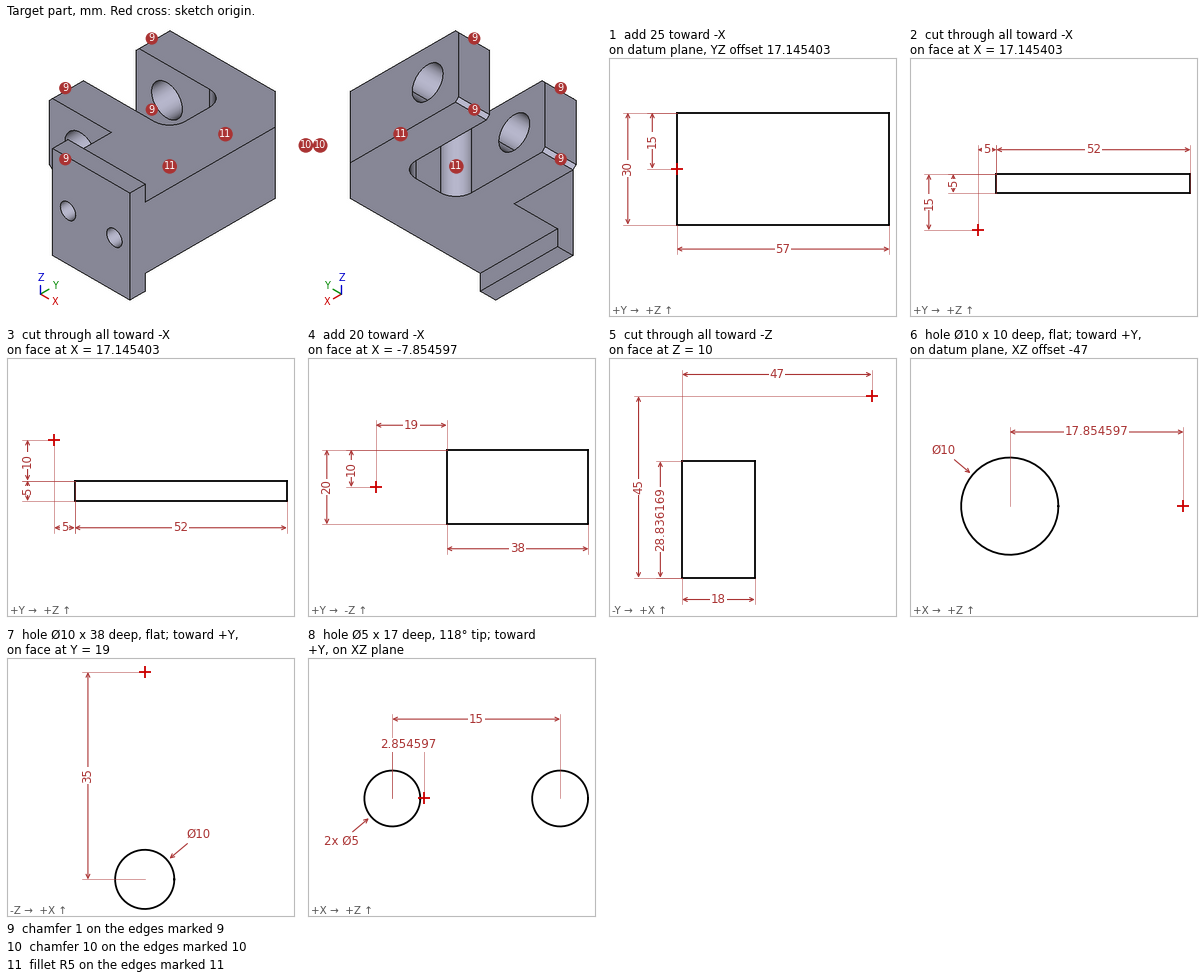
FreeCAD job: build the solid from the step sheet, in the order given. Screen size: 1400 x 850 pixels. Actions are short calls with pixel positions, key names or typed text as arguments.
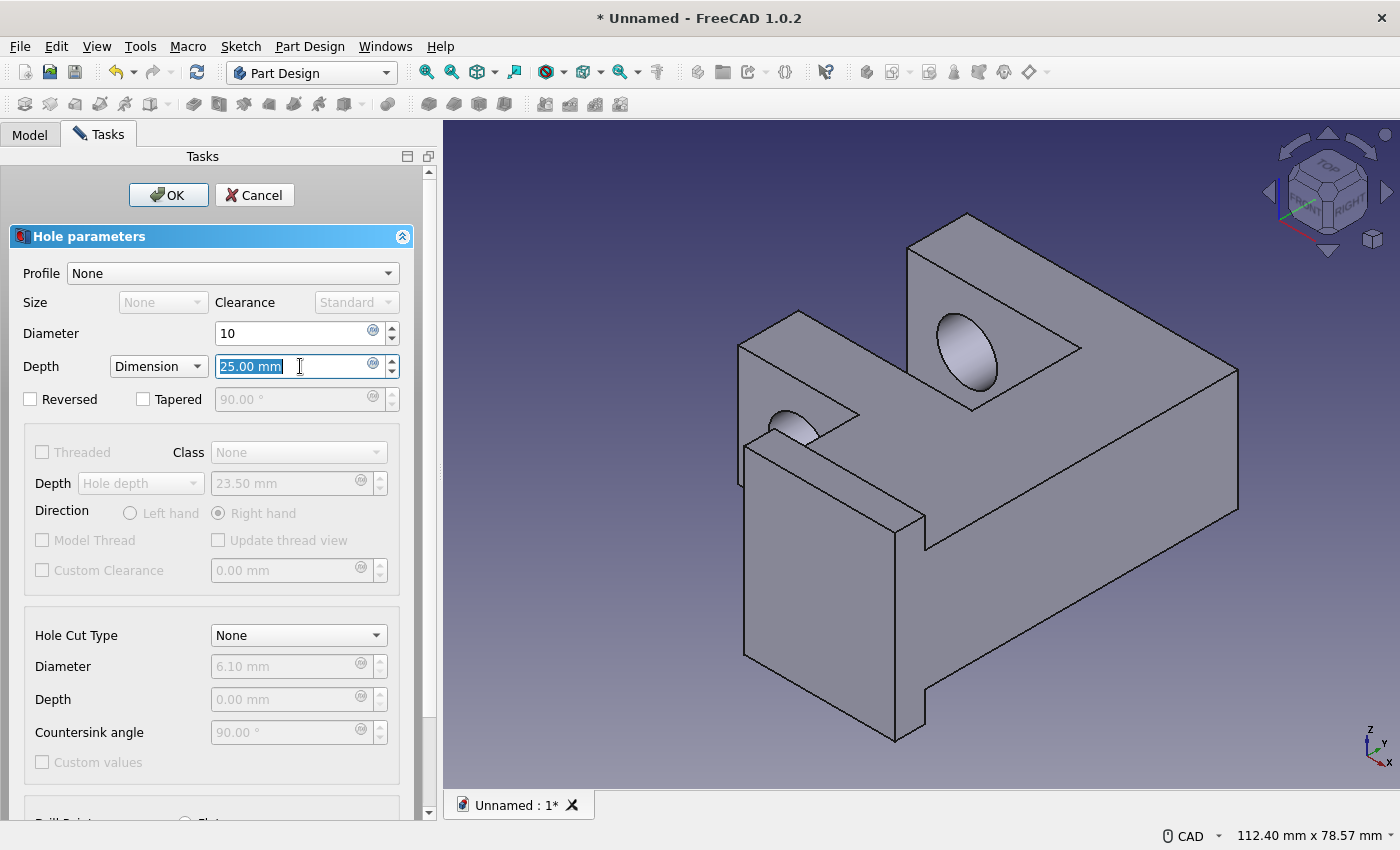
text(38)
key(Tab)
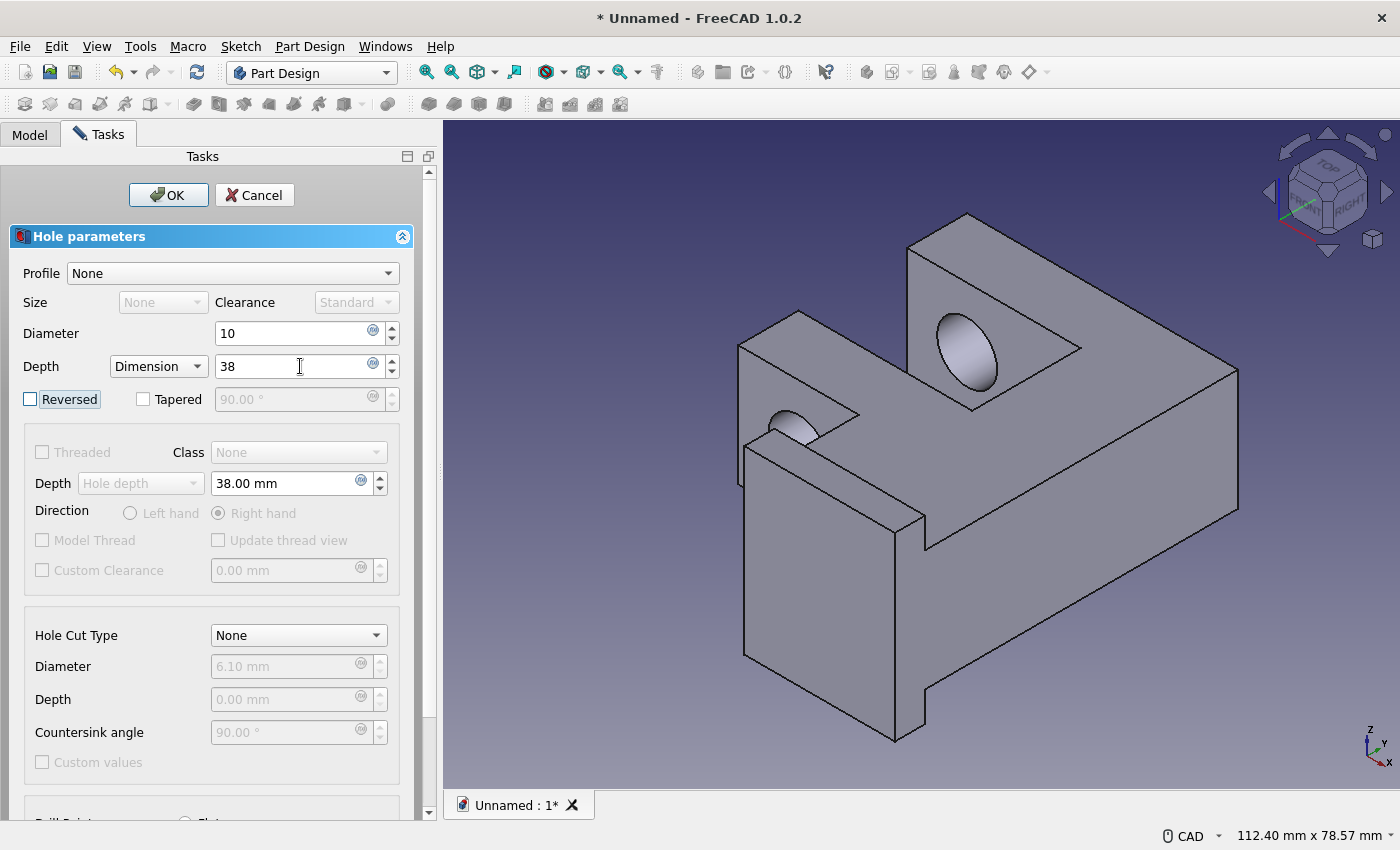
scroll(429, 493, down, 2)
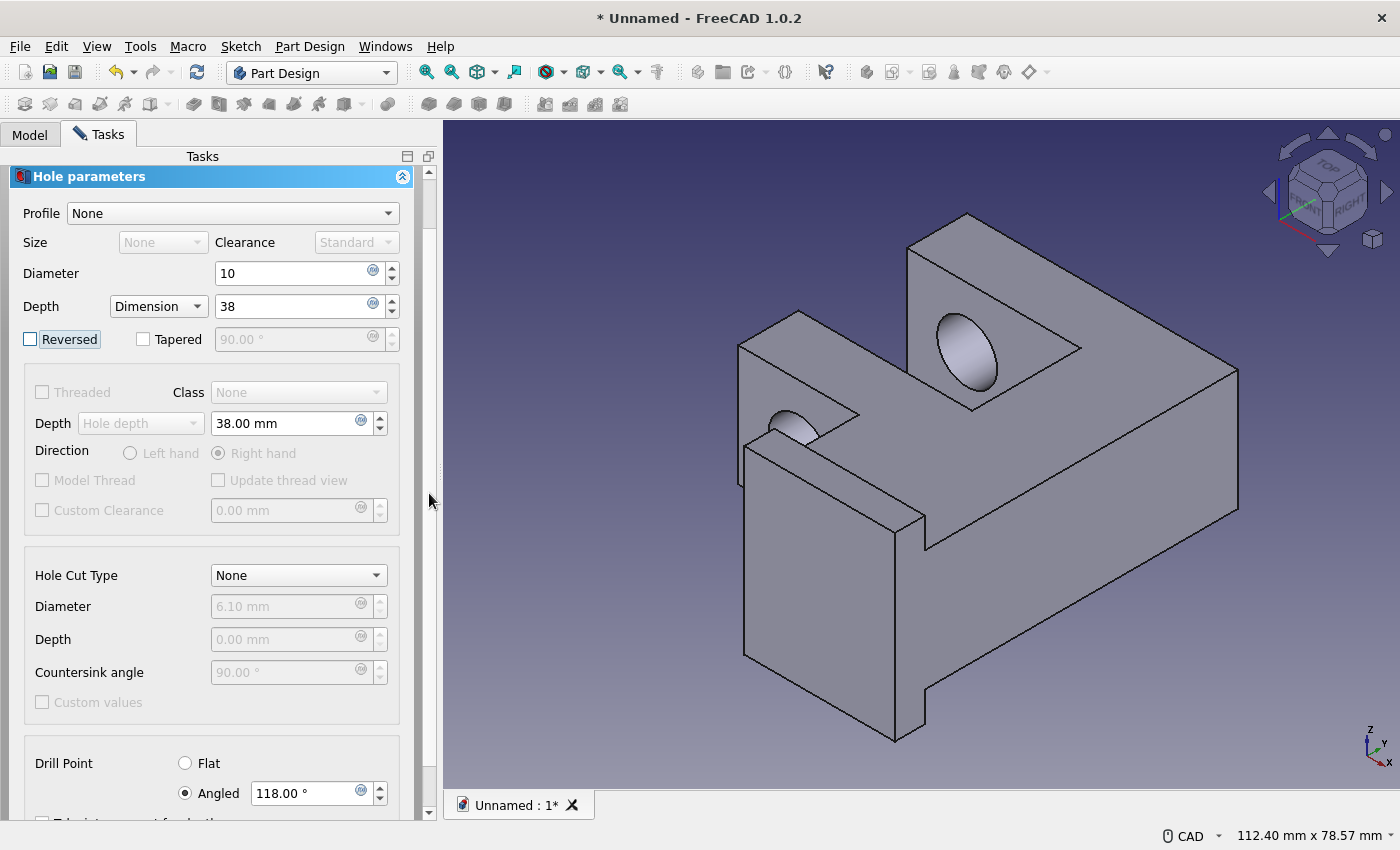
click(186, 713)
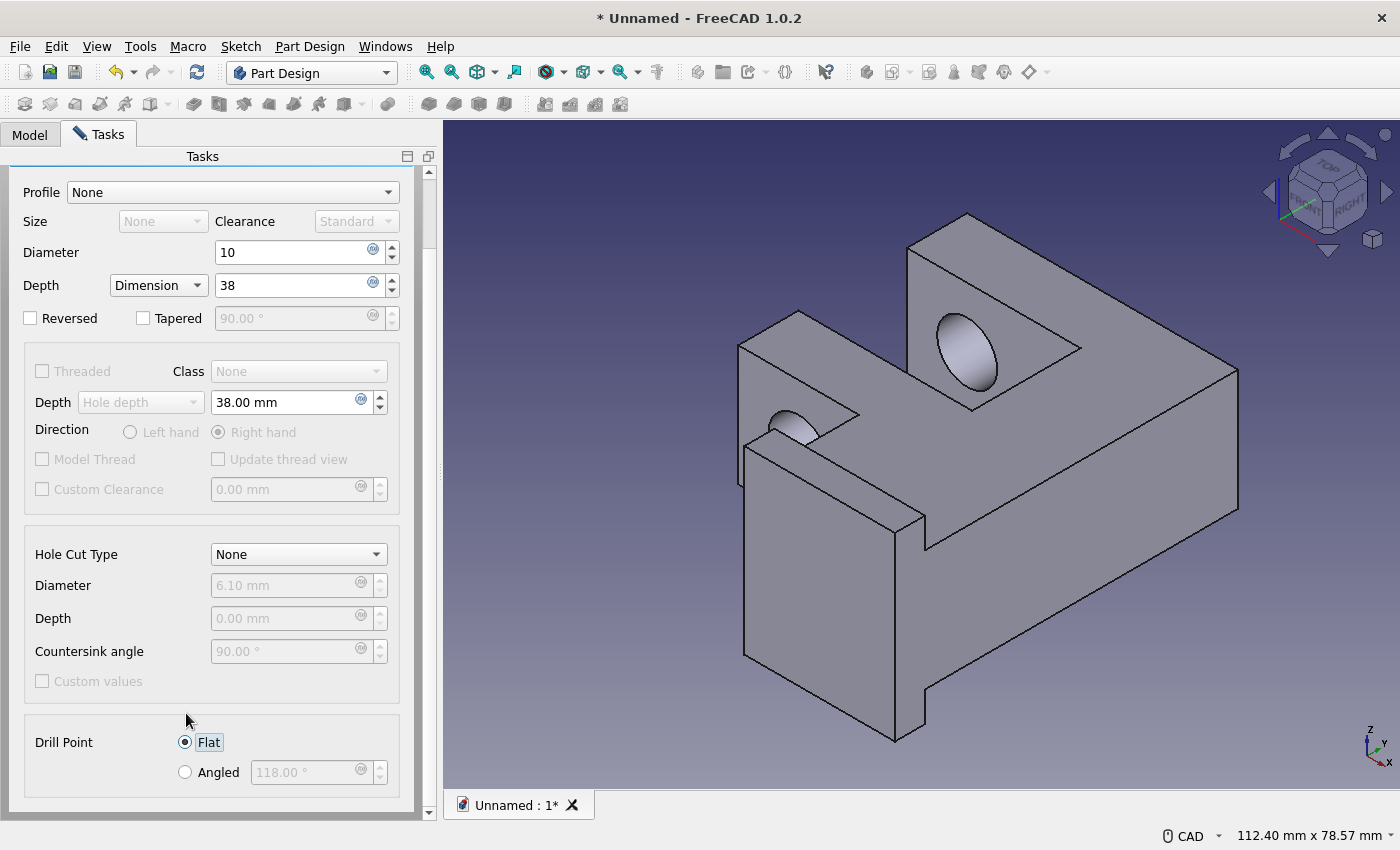
scroll(429, 493, up, 3)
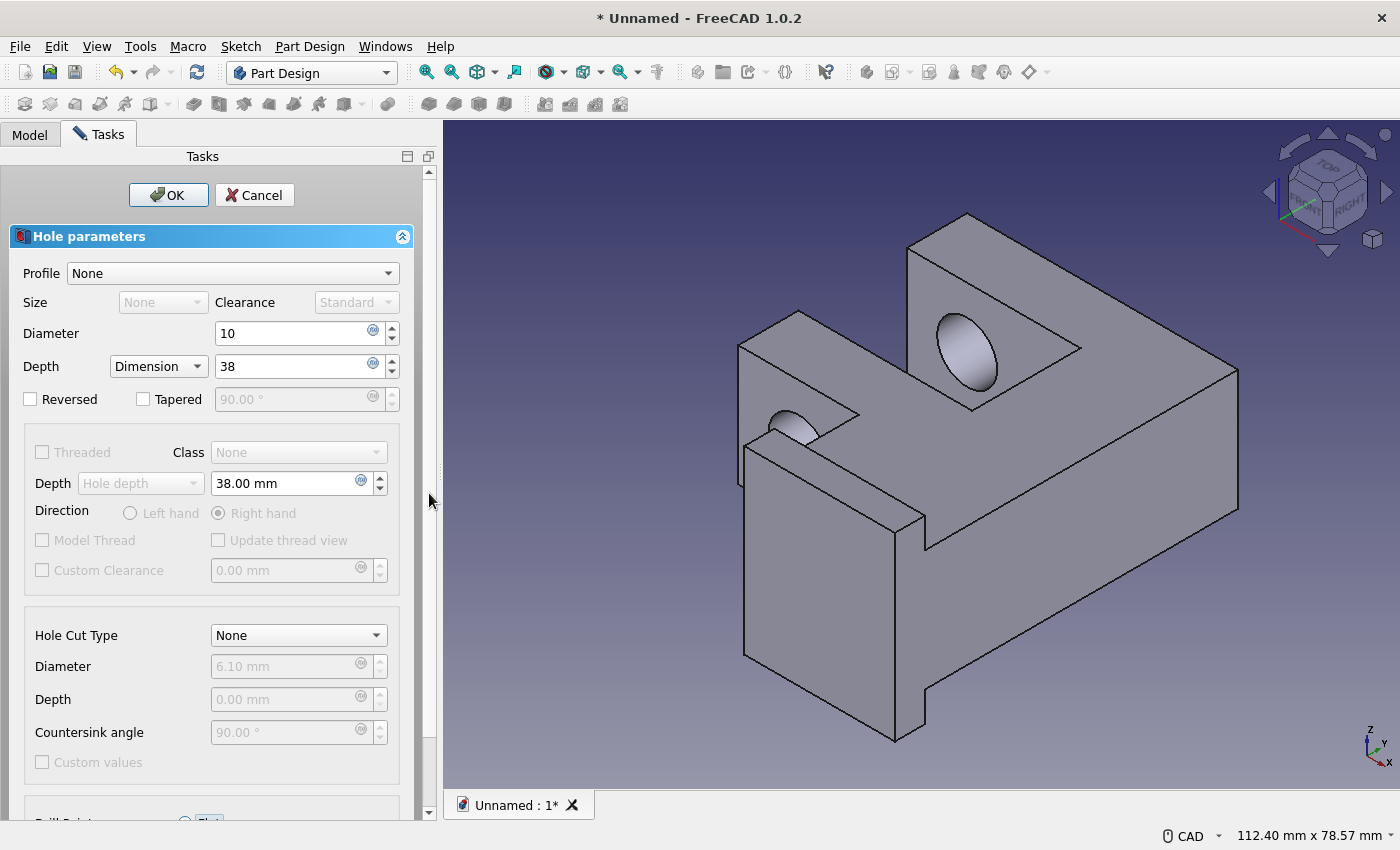
click(169, 195)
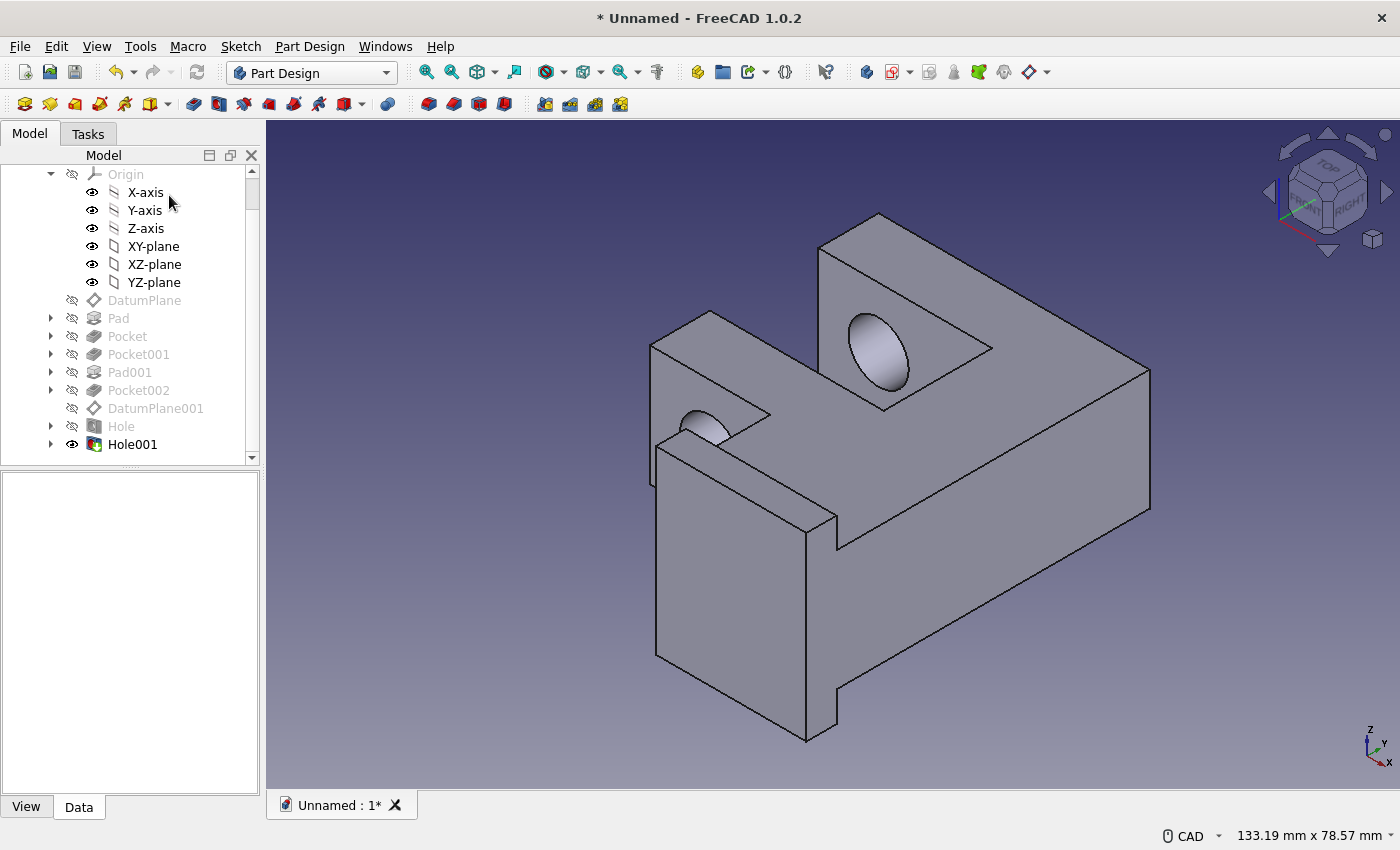
click(892, 72)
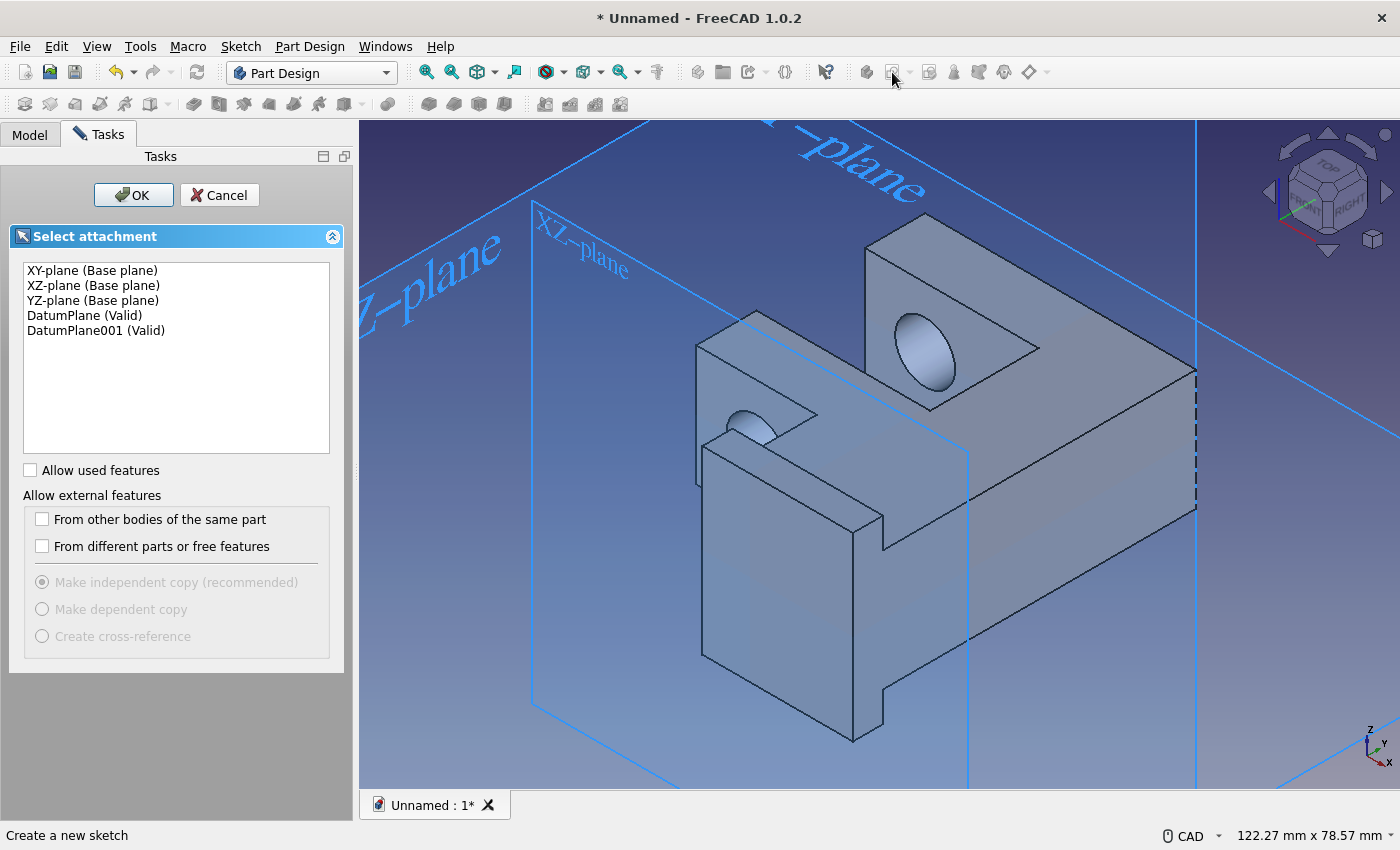
click(84, 286)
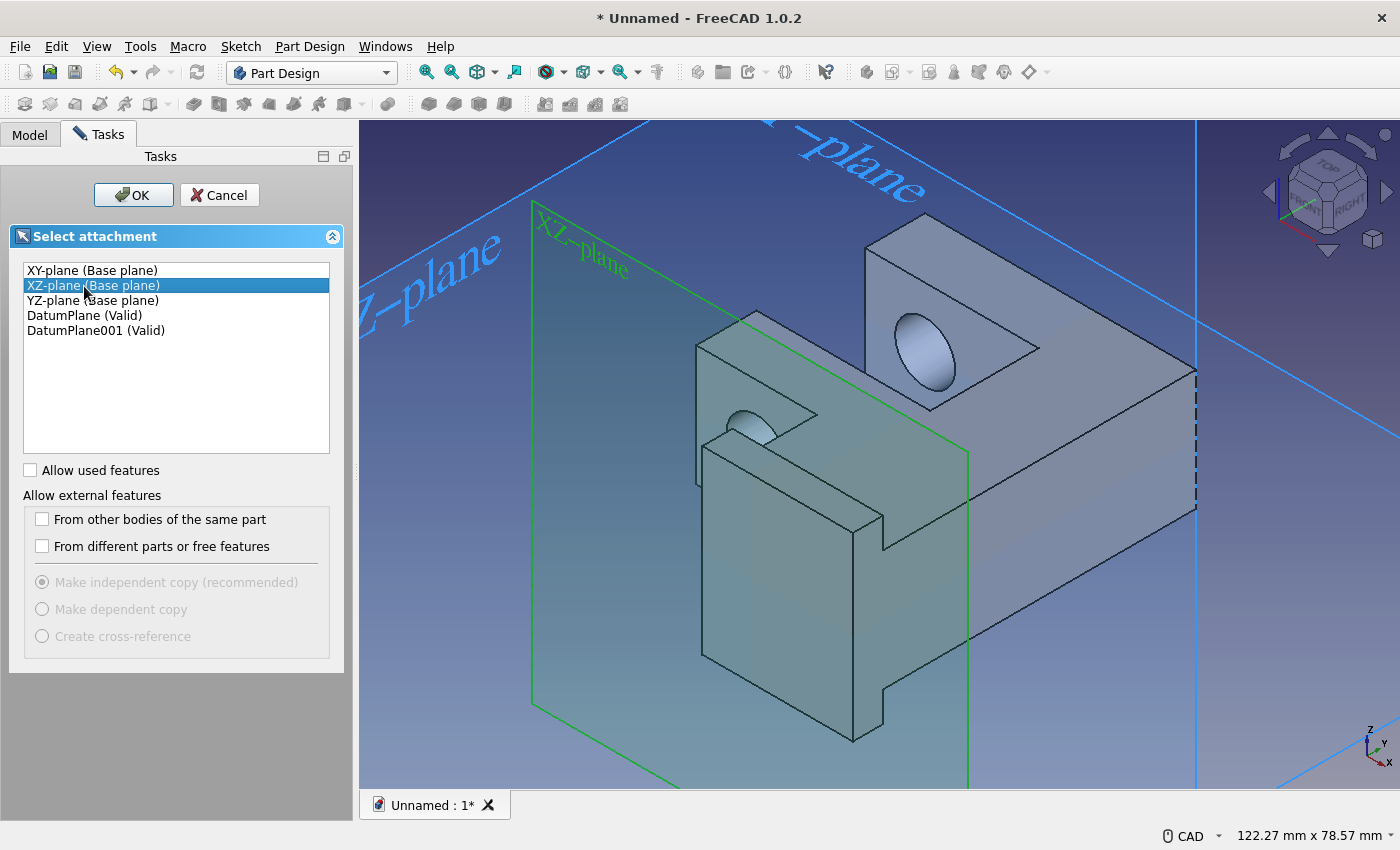
click(134, 195)